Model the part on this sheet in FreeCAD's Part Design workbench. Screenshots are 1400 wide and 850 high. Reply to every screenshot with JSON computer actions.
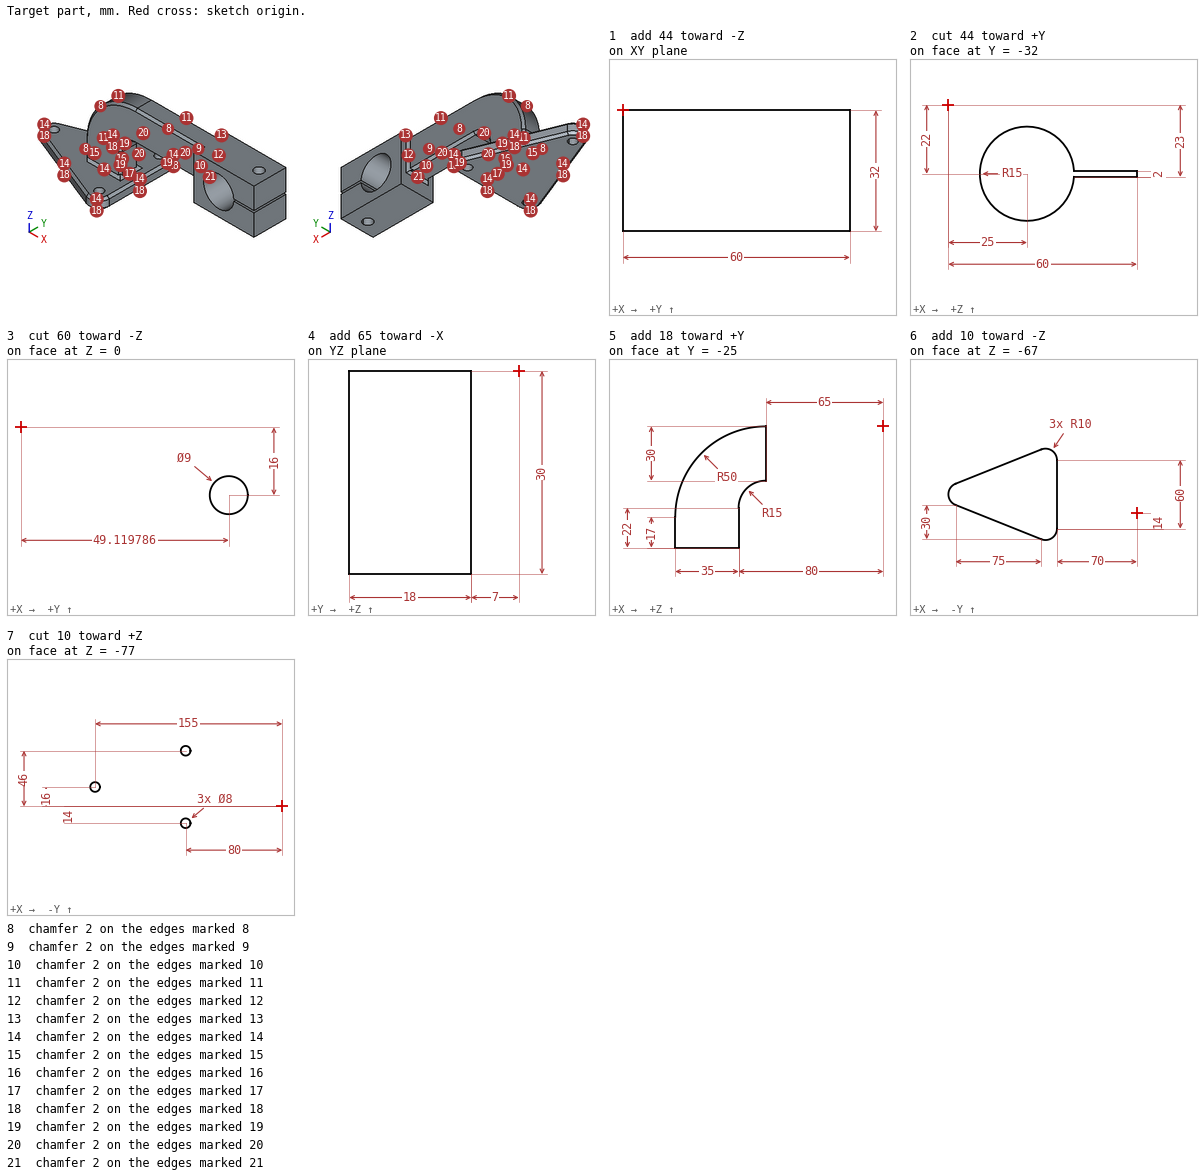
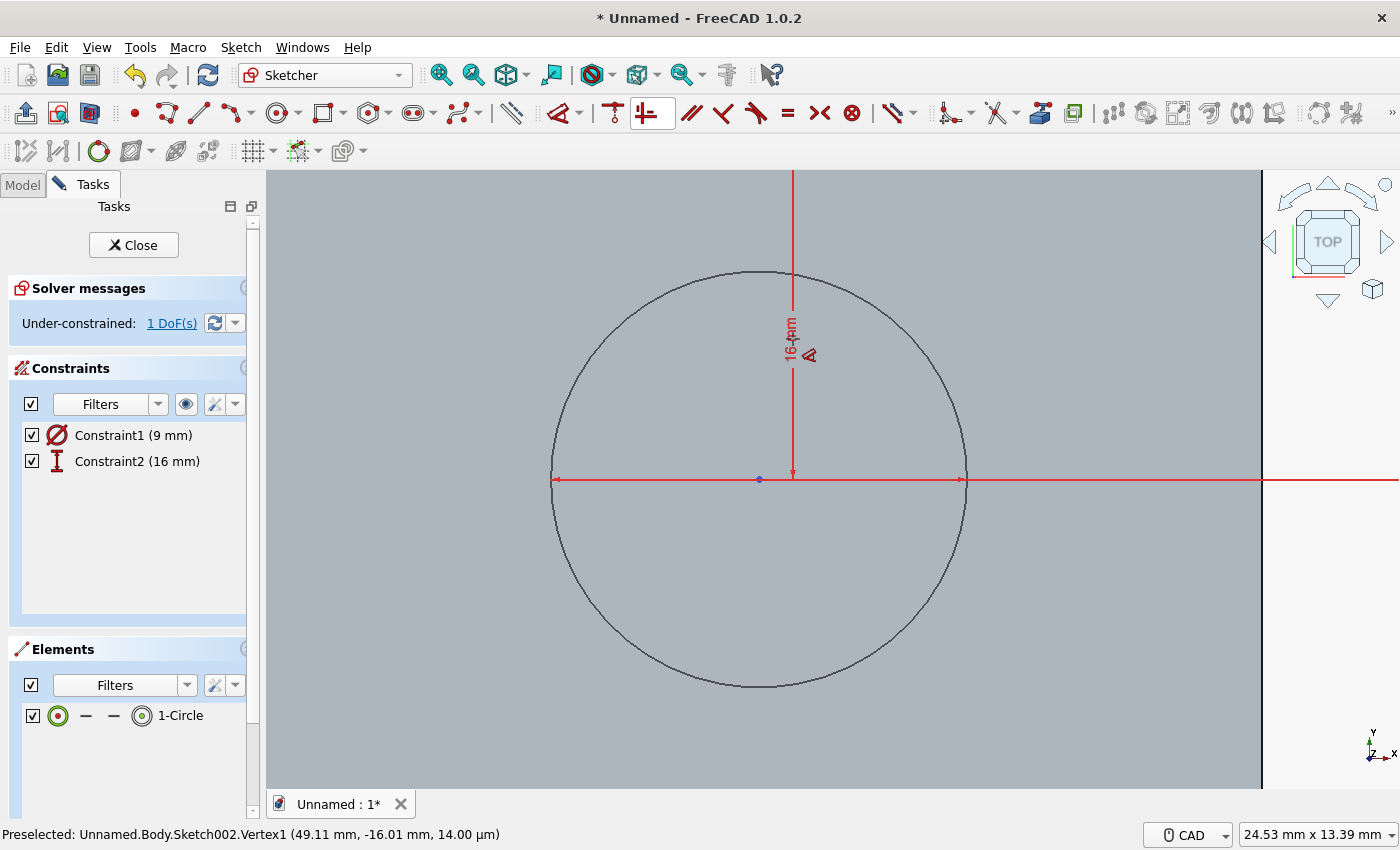
{"action": "left_click", "coordinate": [759, 479]}
{"action": "left_click", "coordinate": [526, 513]}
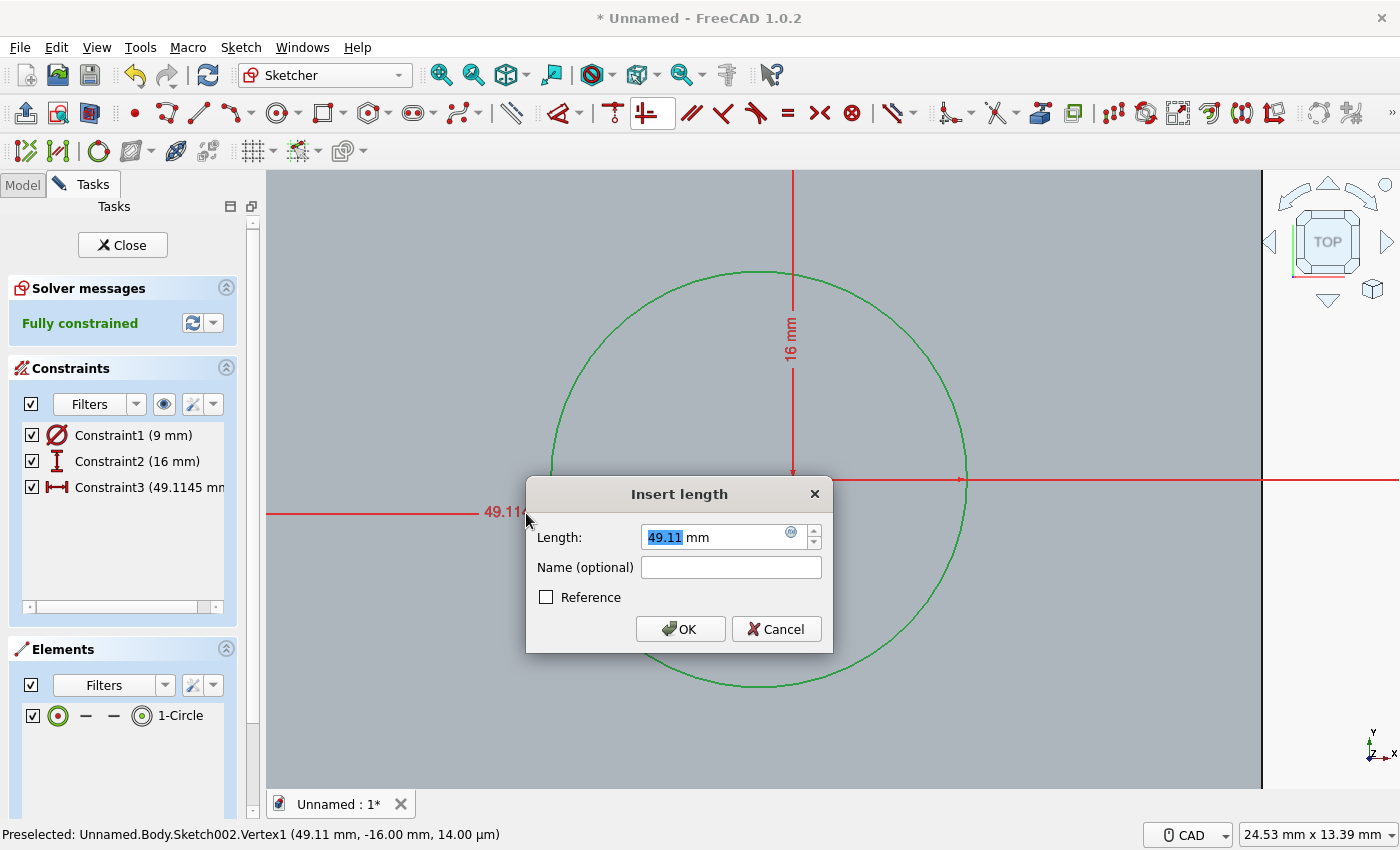
{"action": "type", "text": "49.119786"}
{"action": "key", "text": "Return"}
{"action": "key", "text": "Escape"}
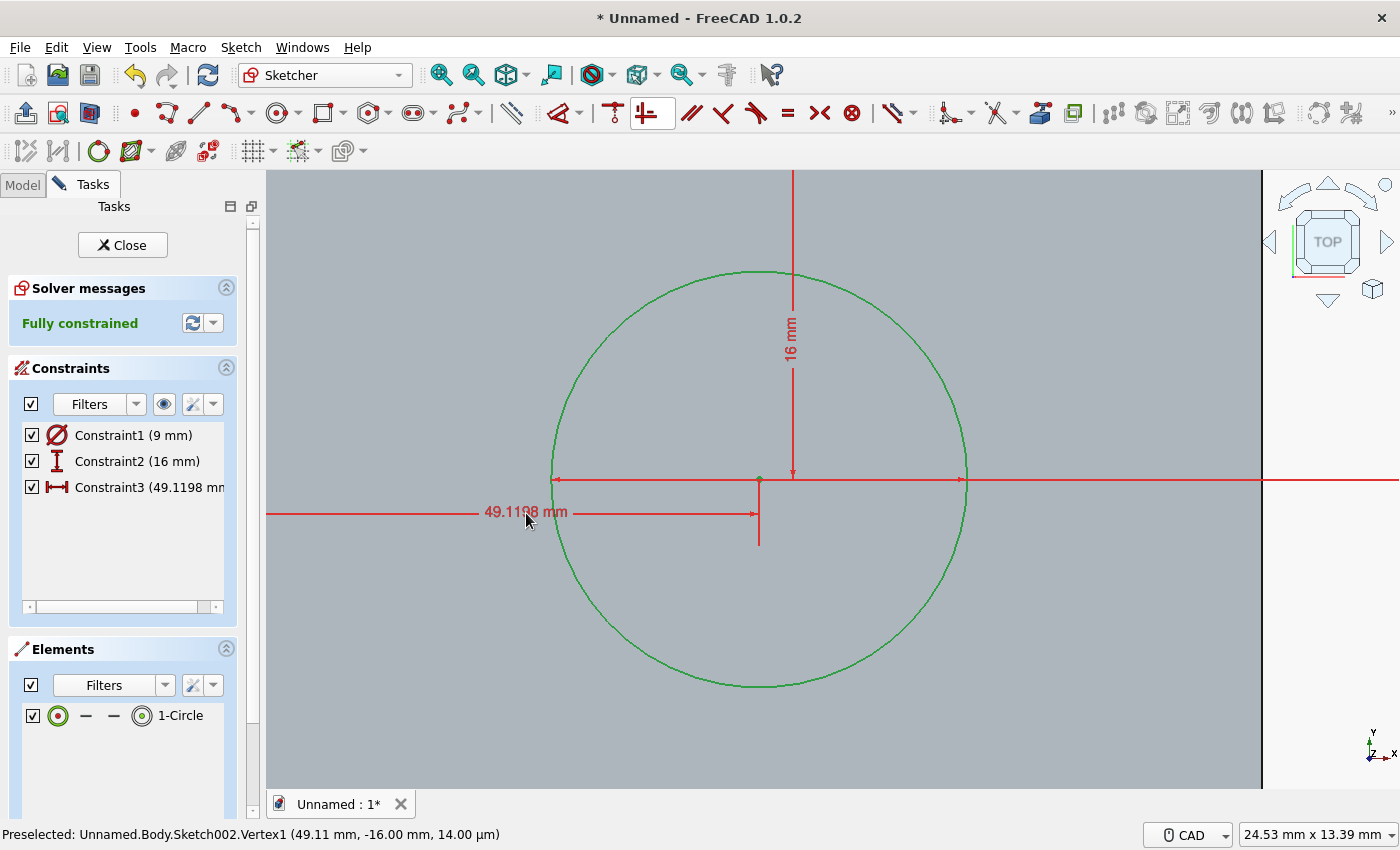
{"action": "left_click", "coordinate": [123, 245]}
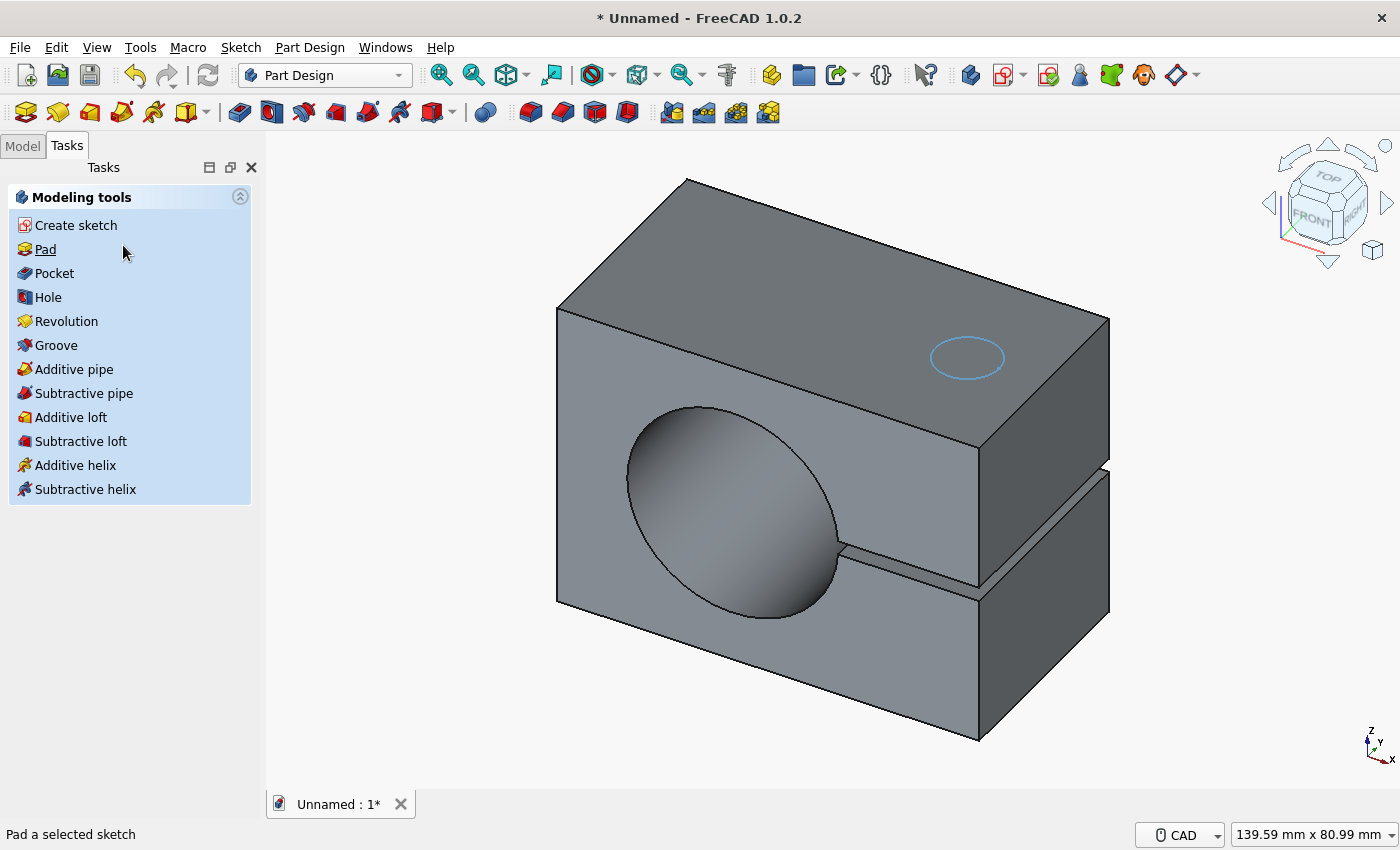
{"action": "left_click", "coordinate": [240, 112]}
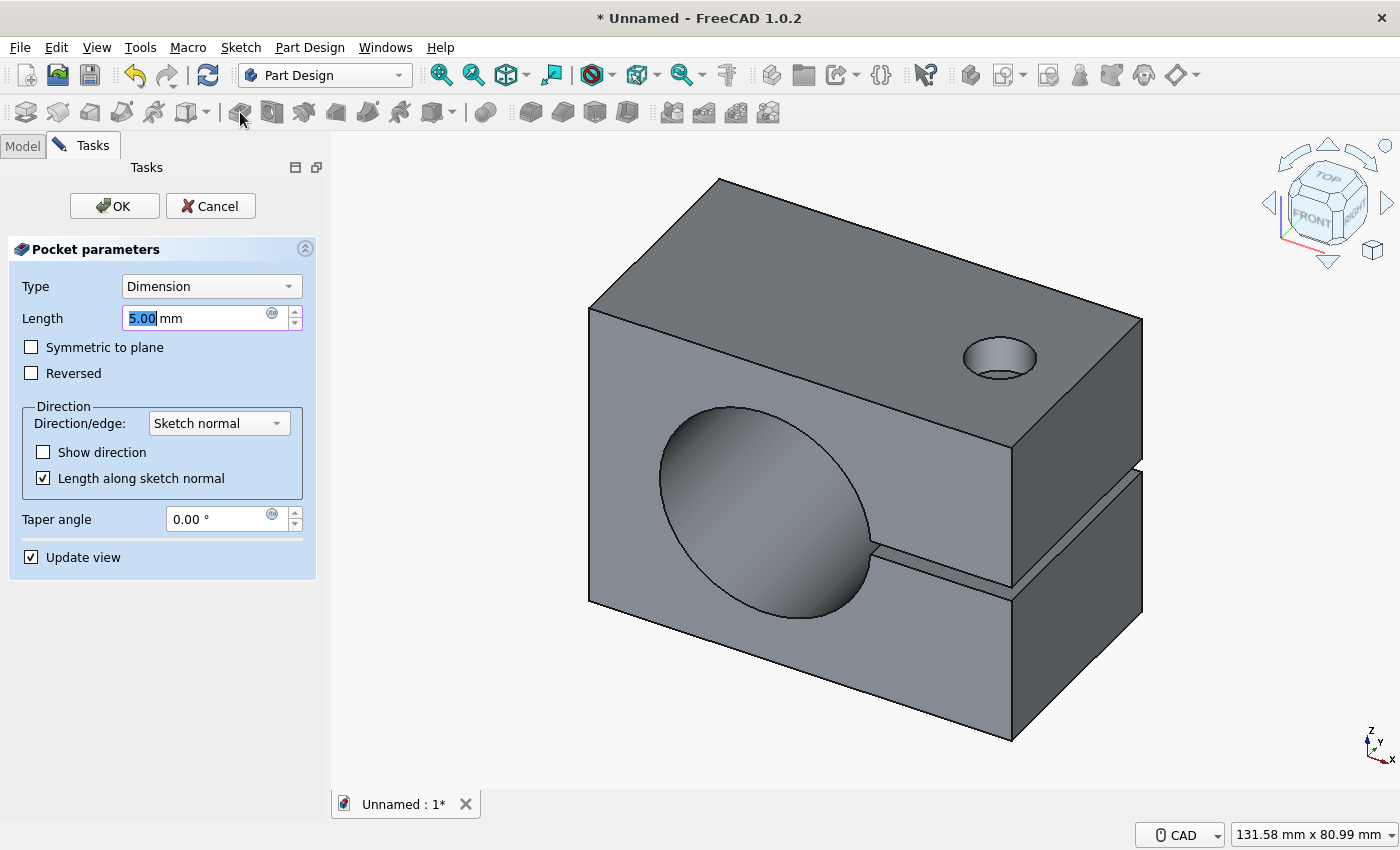
{"action": "type", "text": "60"}
{"action": "key", "text": "Tab"}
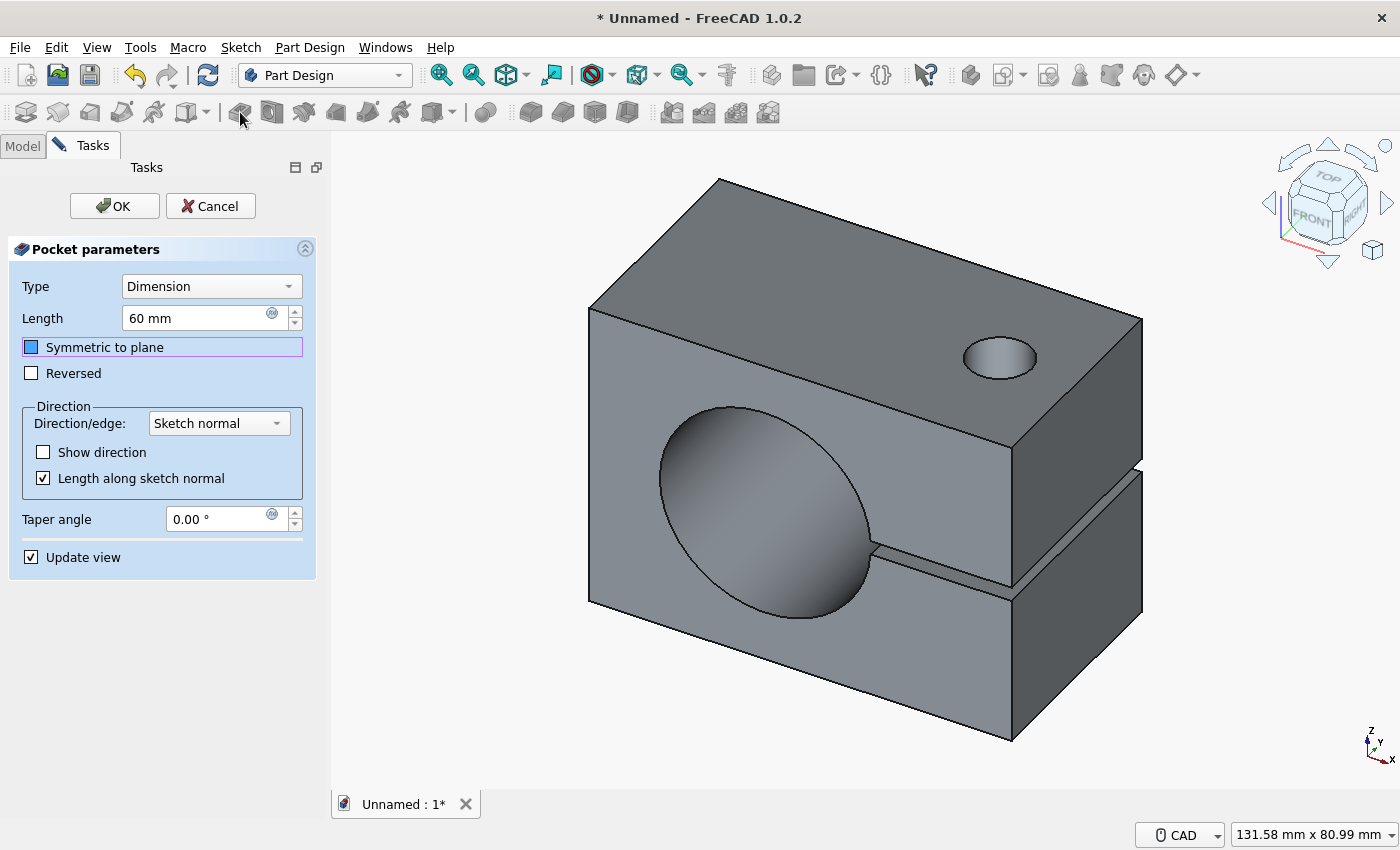
{"action": "left_click", "coordinate": [115, 206]}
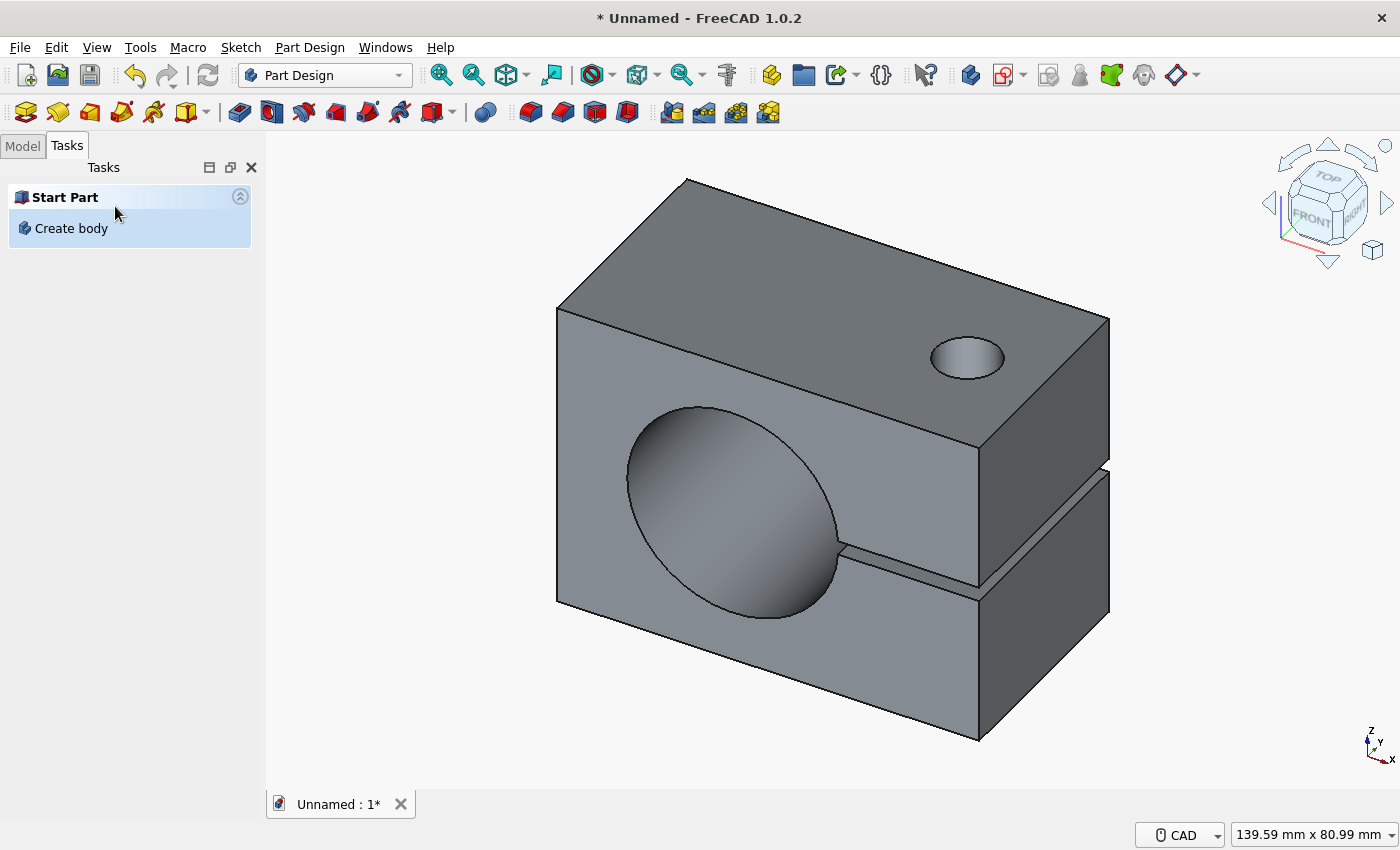
{"action": "left_click", "coordinate": [1004, 76]}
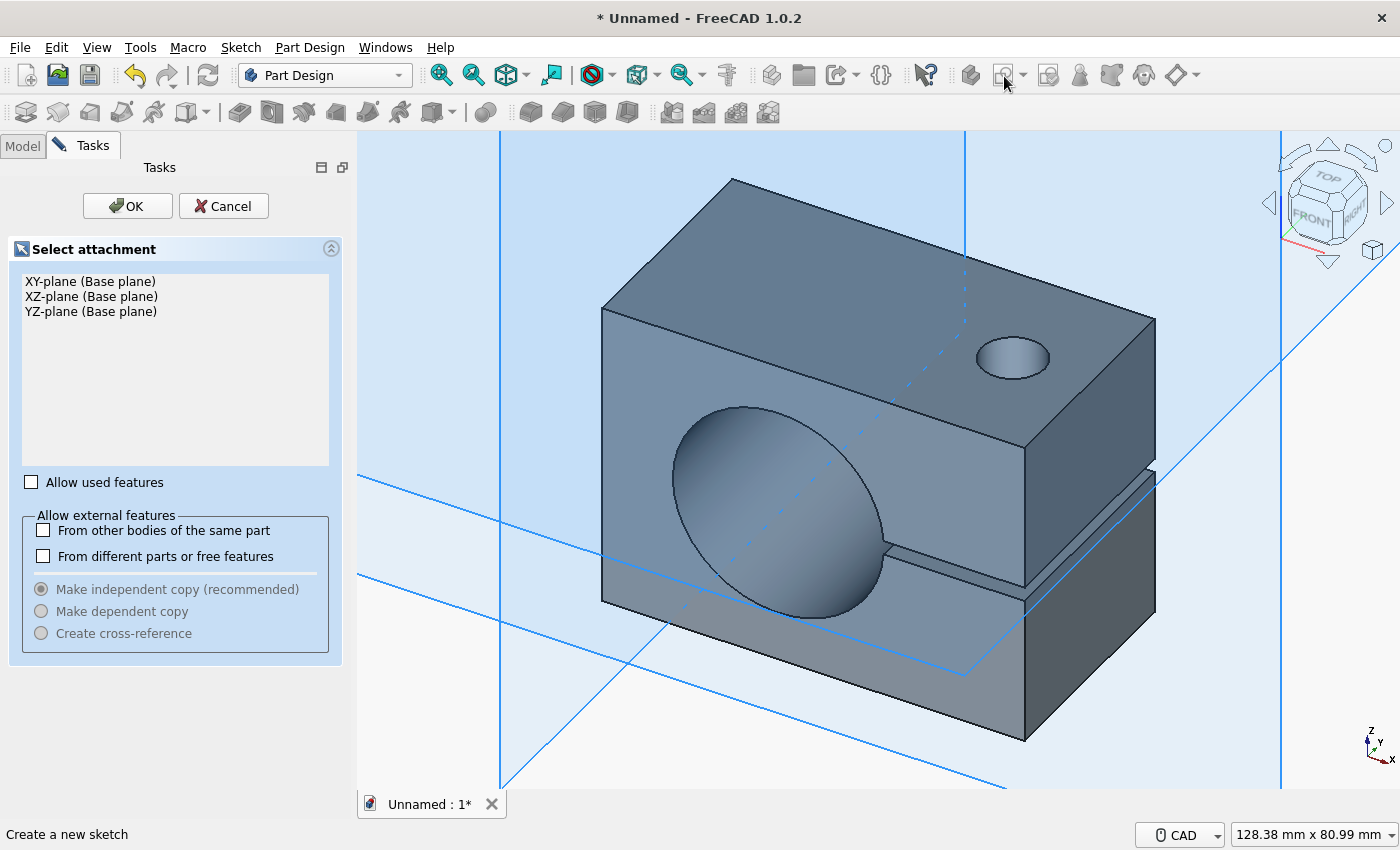
{"action": "left_click", "coordinate": [82, 312]}